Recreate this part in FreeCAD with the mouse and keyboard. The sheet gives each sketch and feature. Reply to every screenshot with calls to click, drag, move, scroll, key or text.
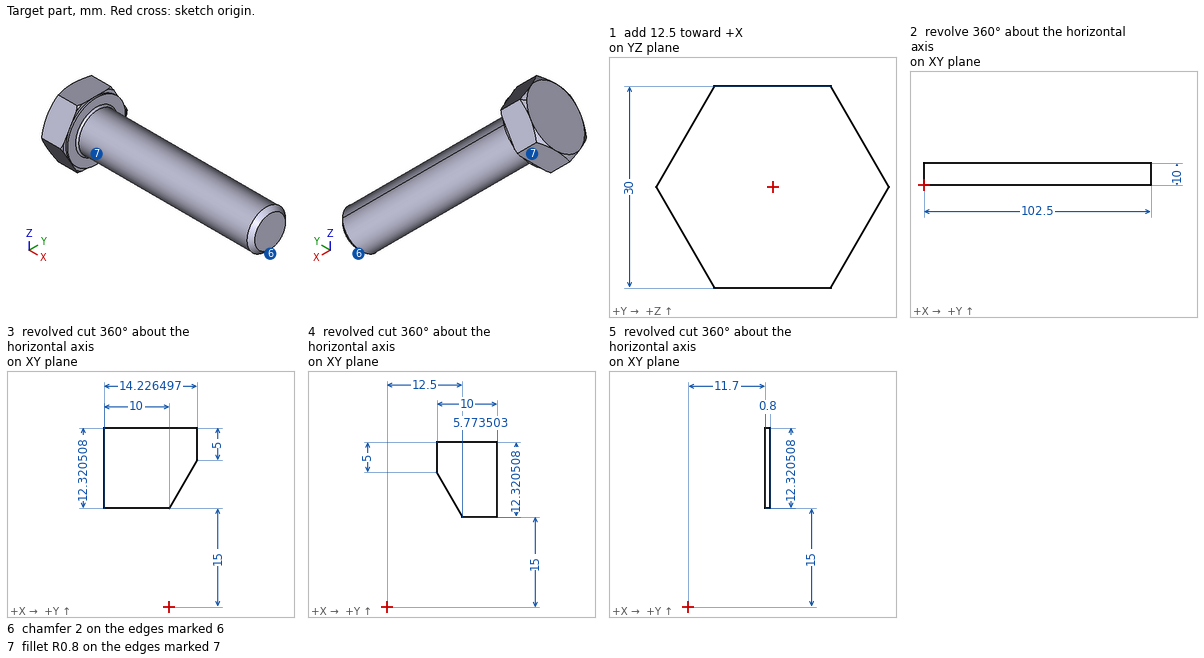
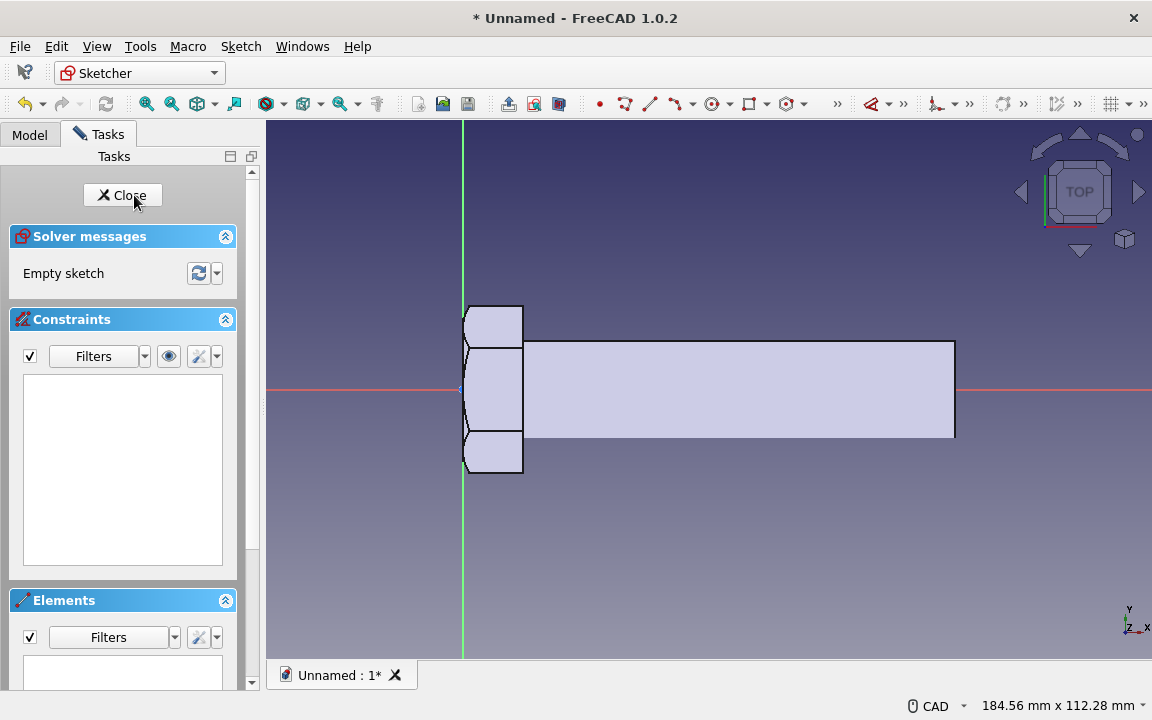
click(559, 104)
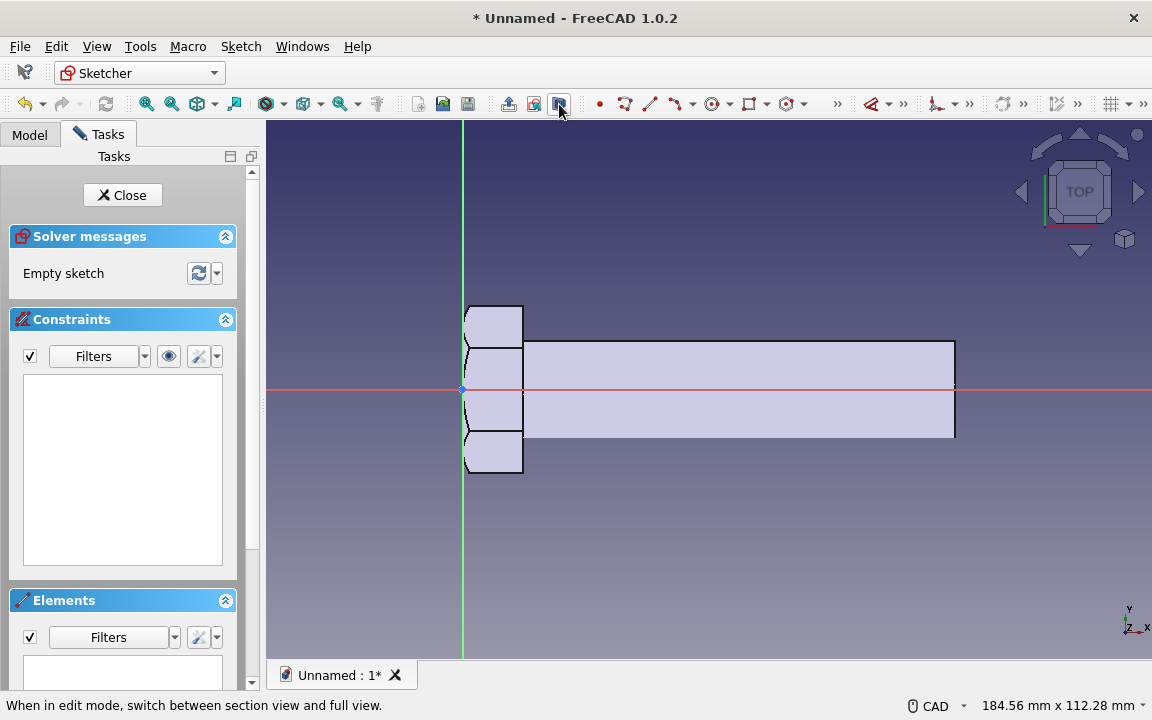
scroll(429, 286, up, 5)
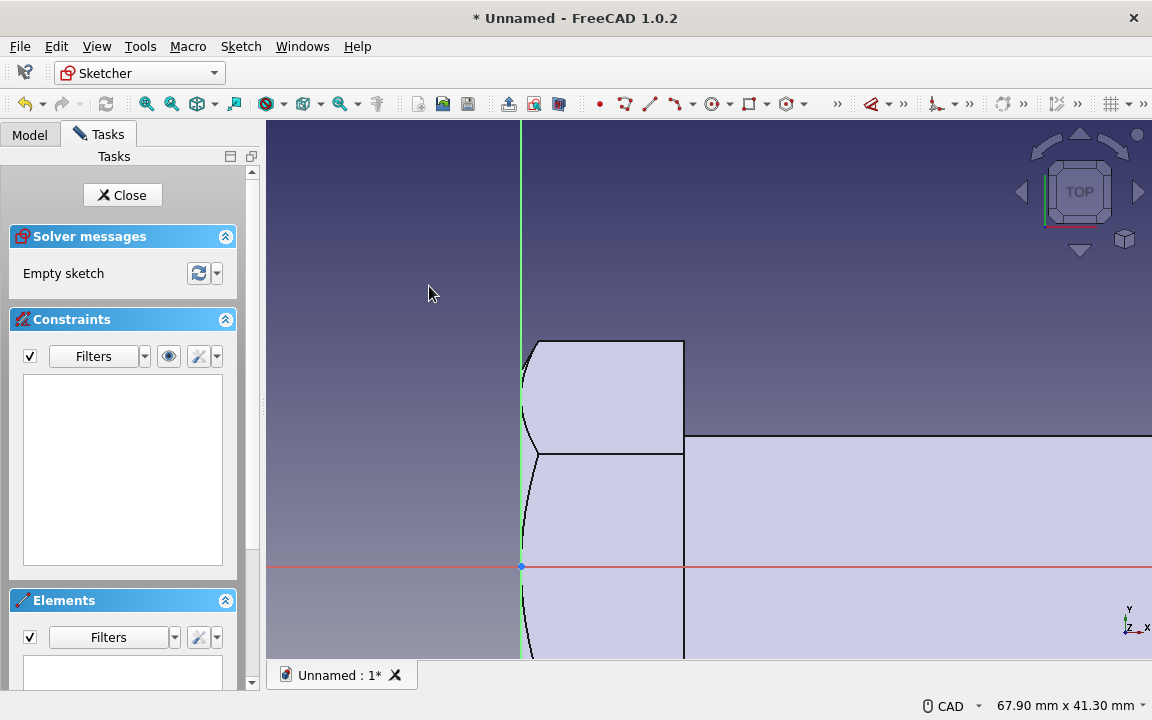
key(g)
key(m)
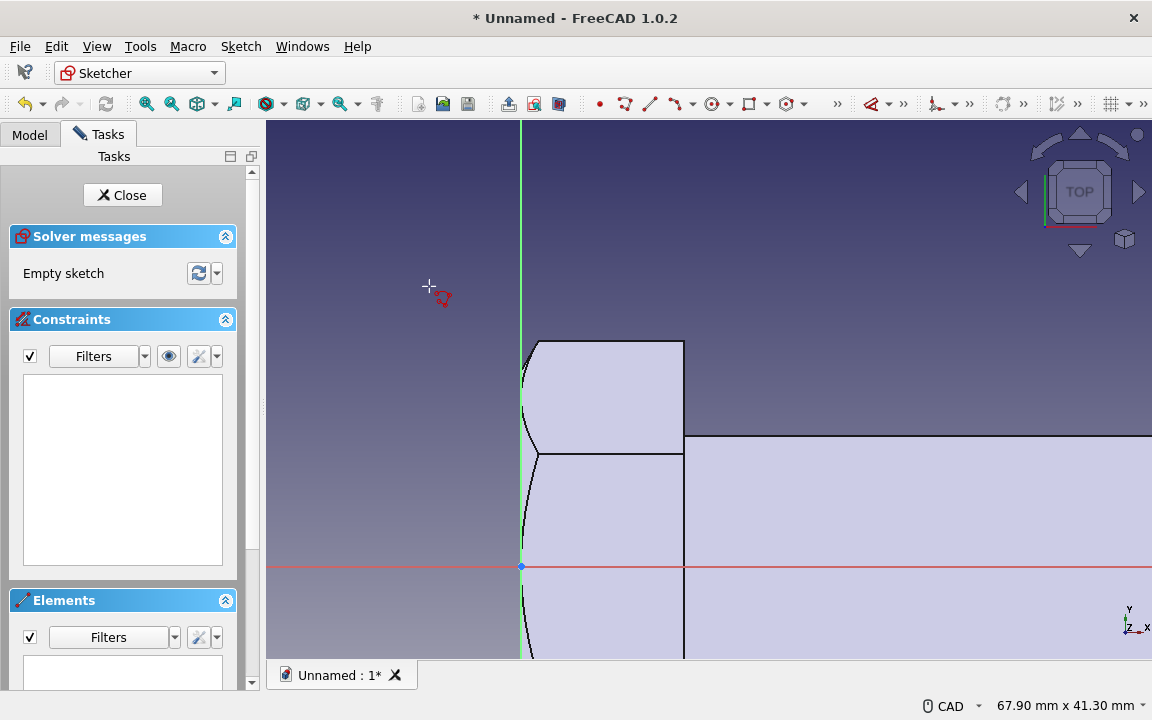
click(684, 371)
click(759, 371)
click(759, 210)
click(629, 210)
click(629, 276)
click(684, 372)
key(Escape)
key(Escape)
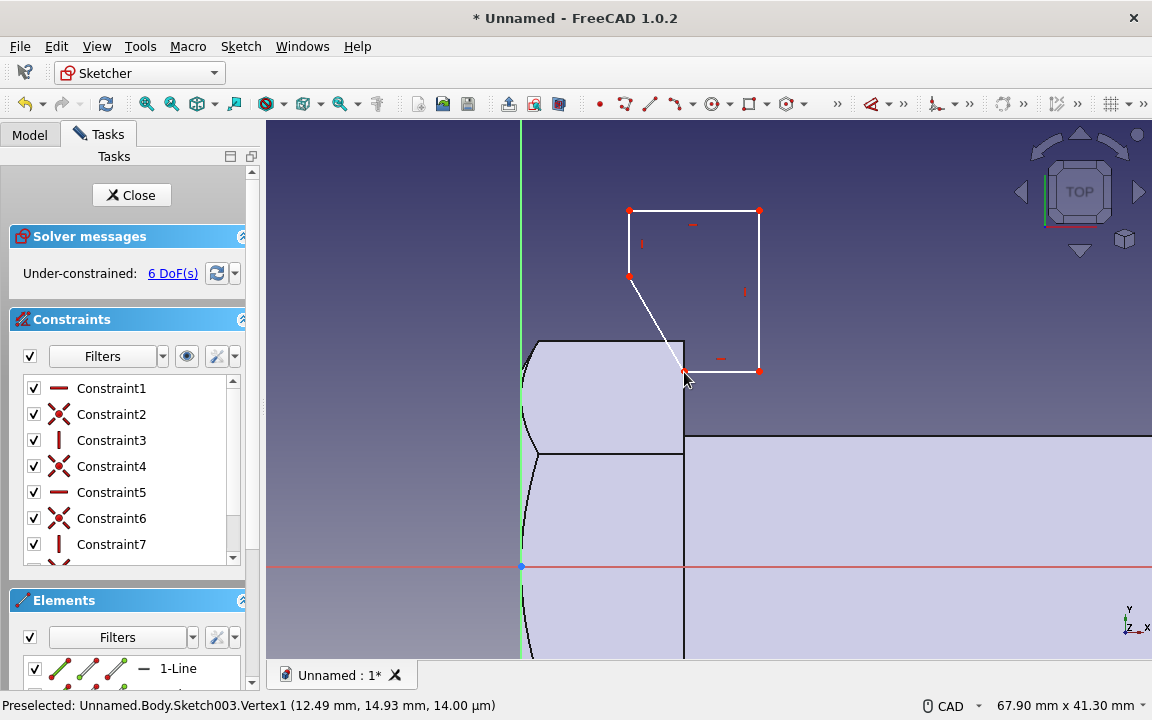
click(629, 231)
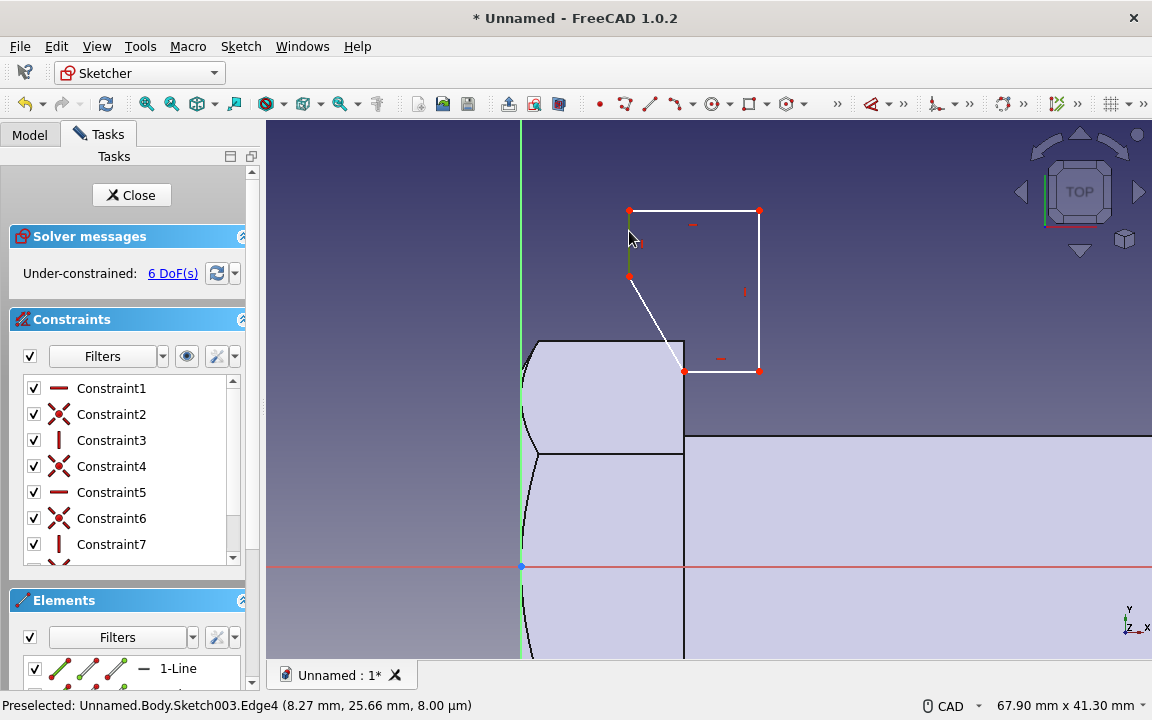
click(888, 104)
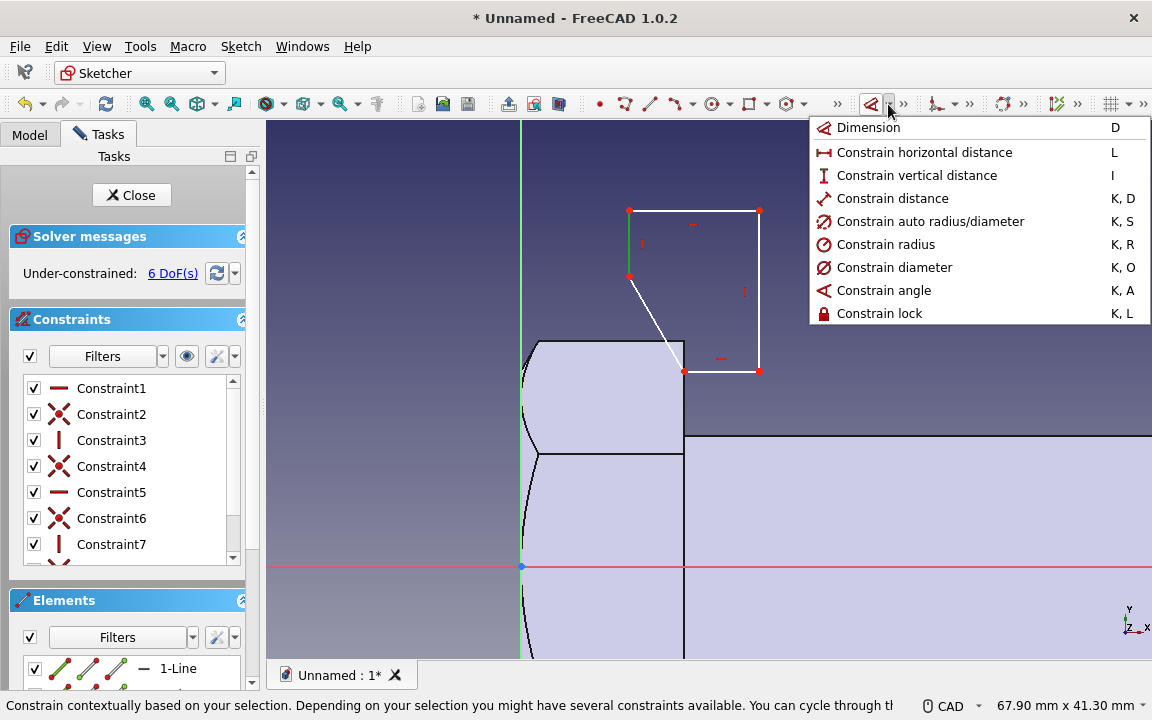
click(980, 176)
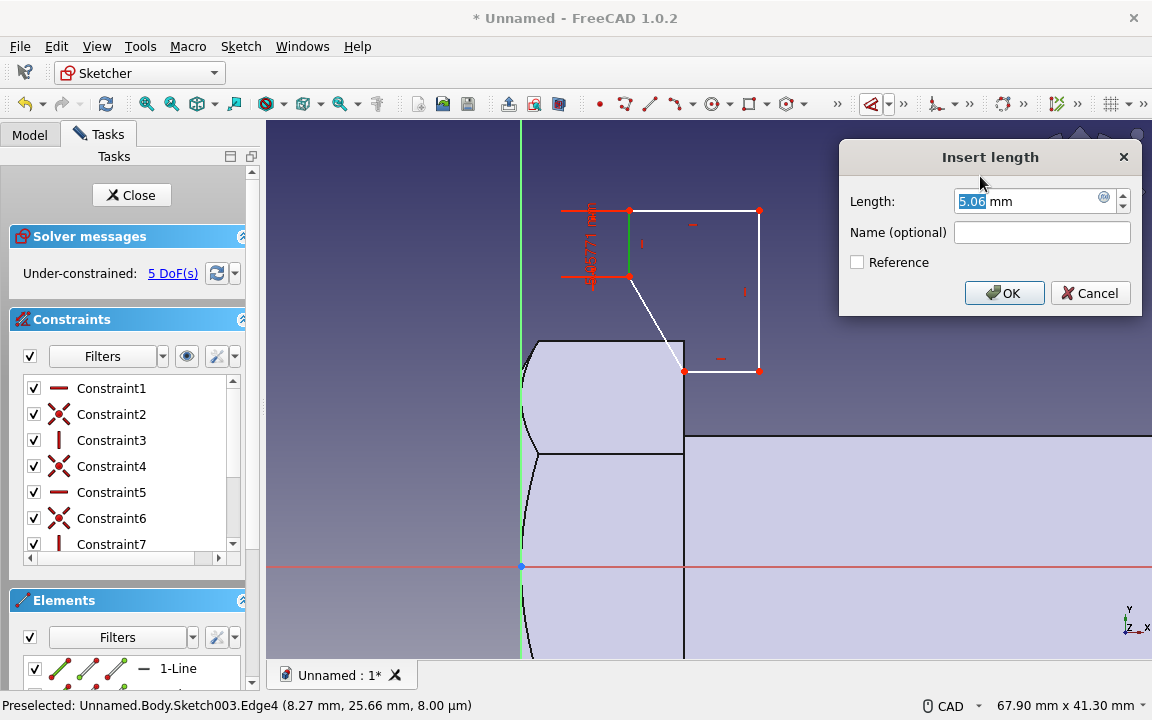
text(5)
key(Return)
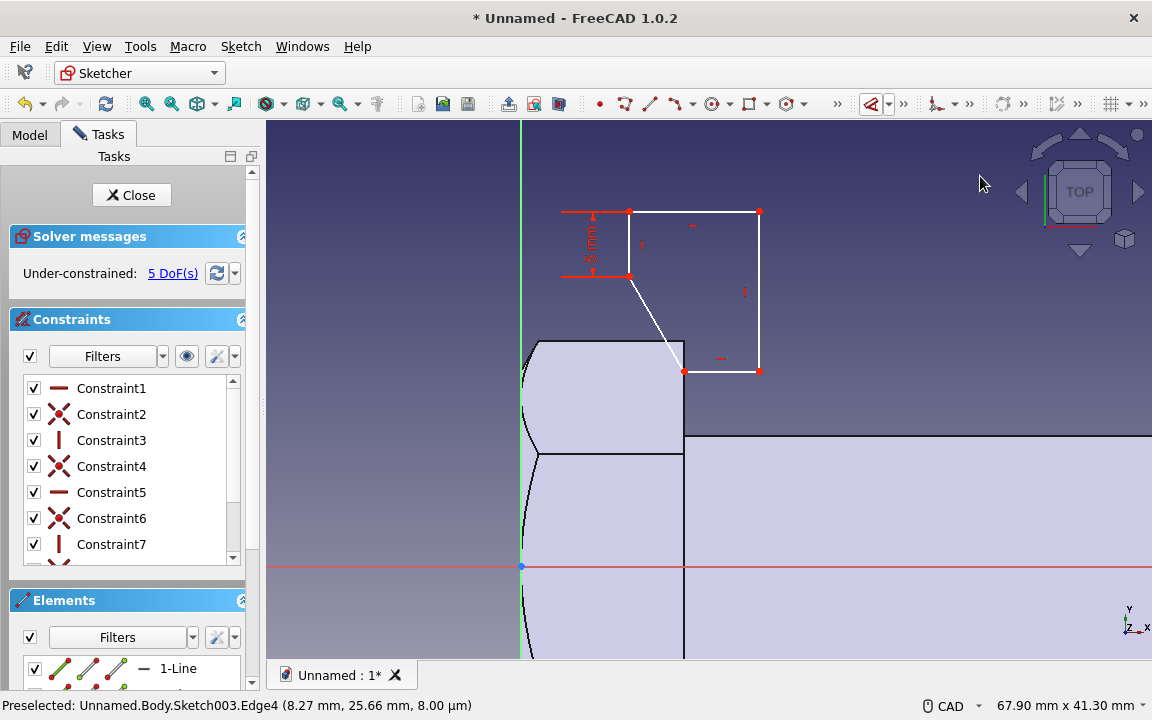
click(720, 212)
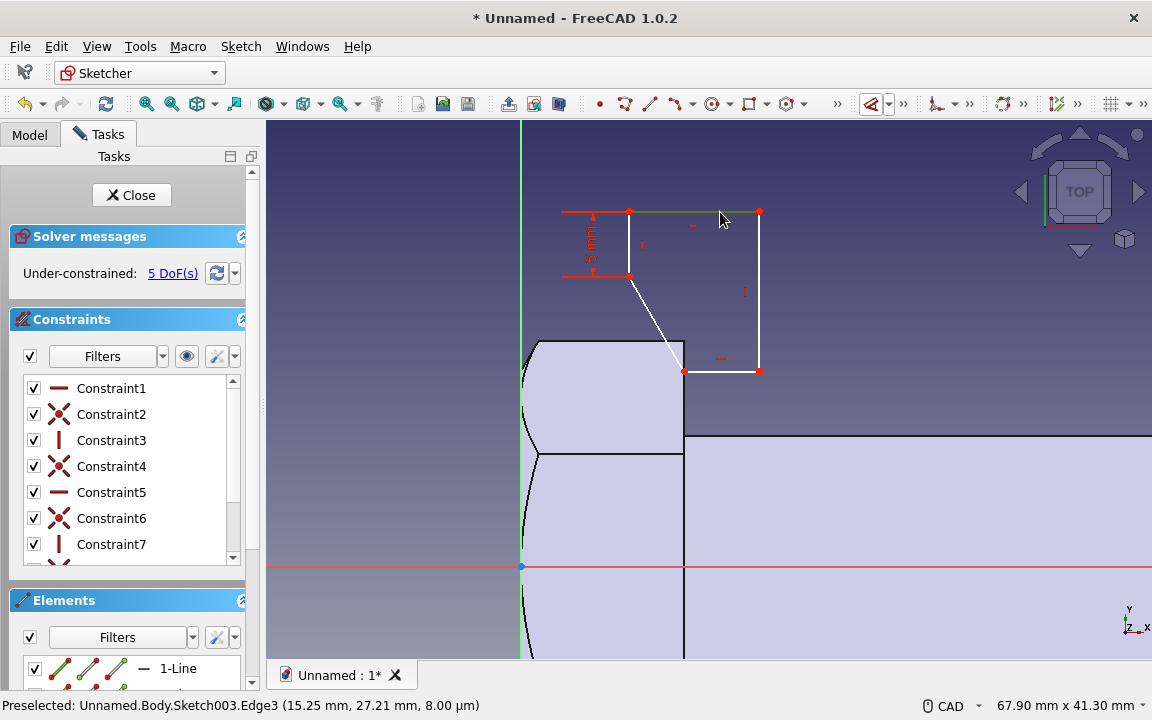
key(l)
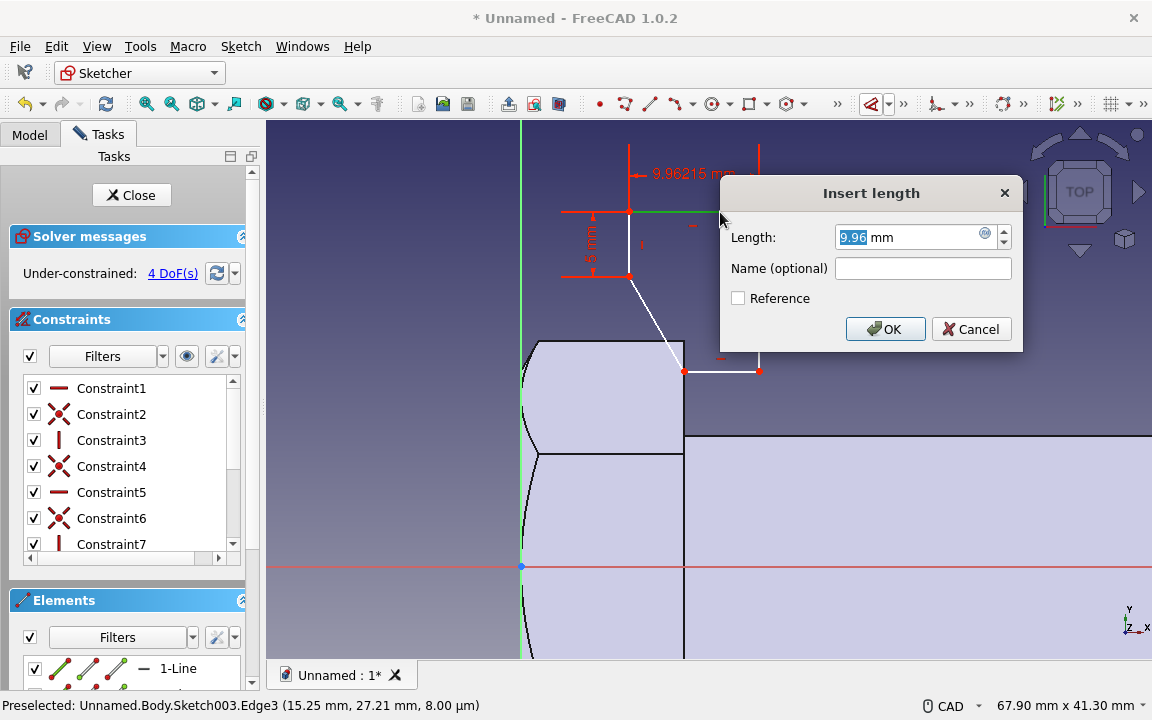
text(10)
key(Return)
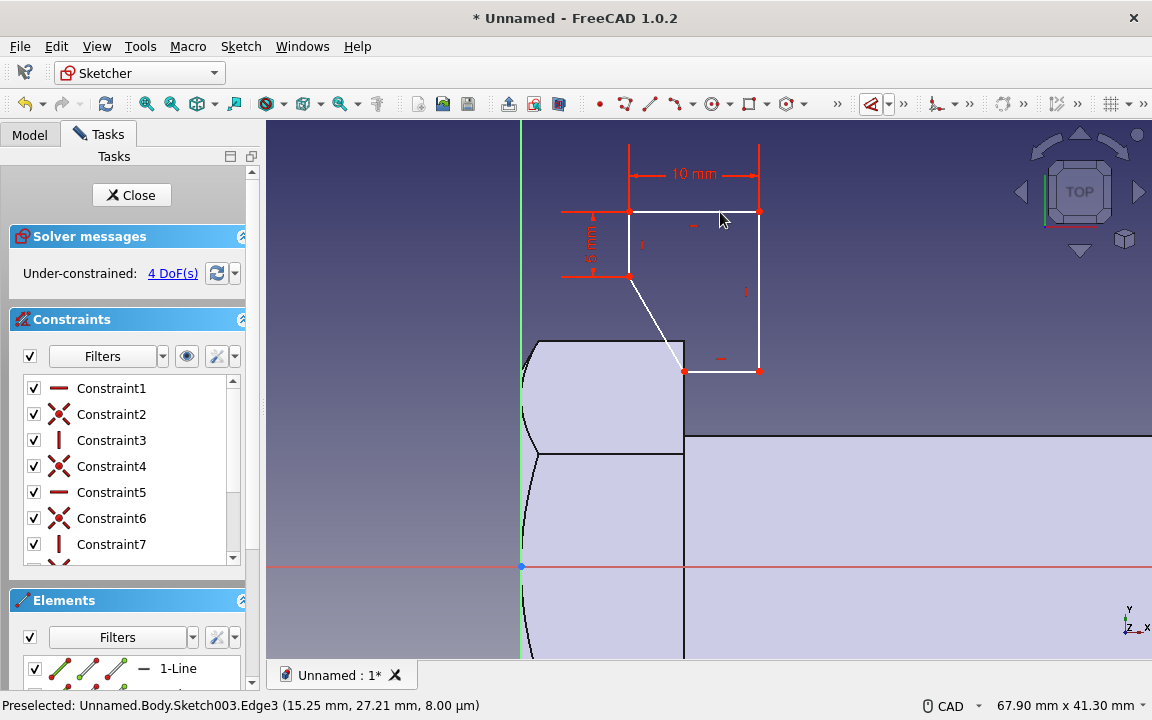
click(684, 372)